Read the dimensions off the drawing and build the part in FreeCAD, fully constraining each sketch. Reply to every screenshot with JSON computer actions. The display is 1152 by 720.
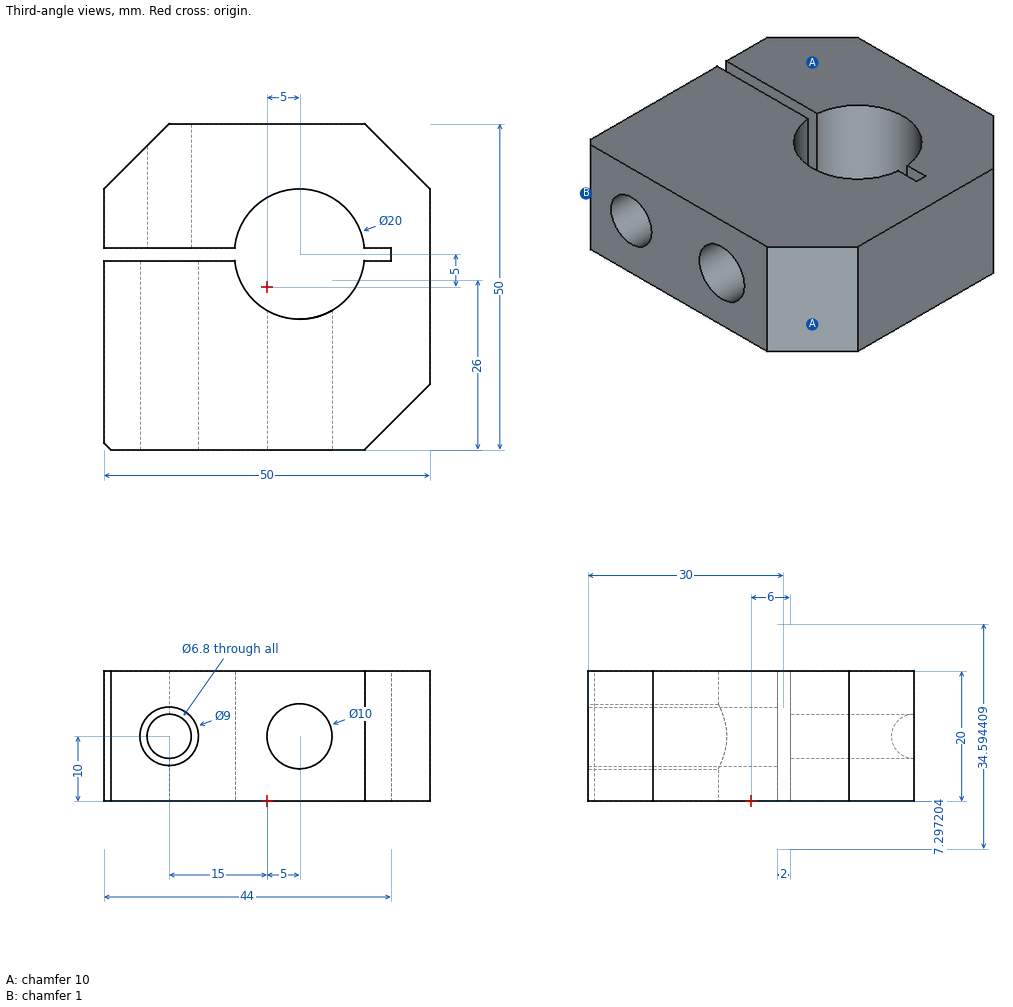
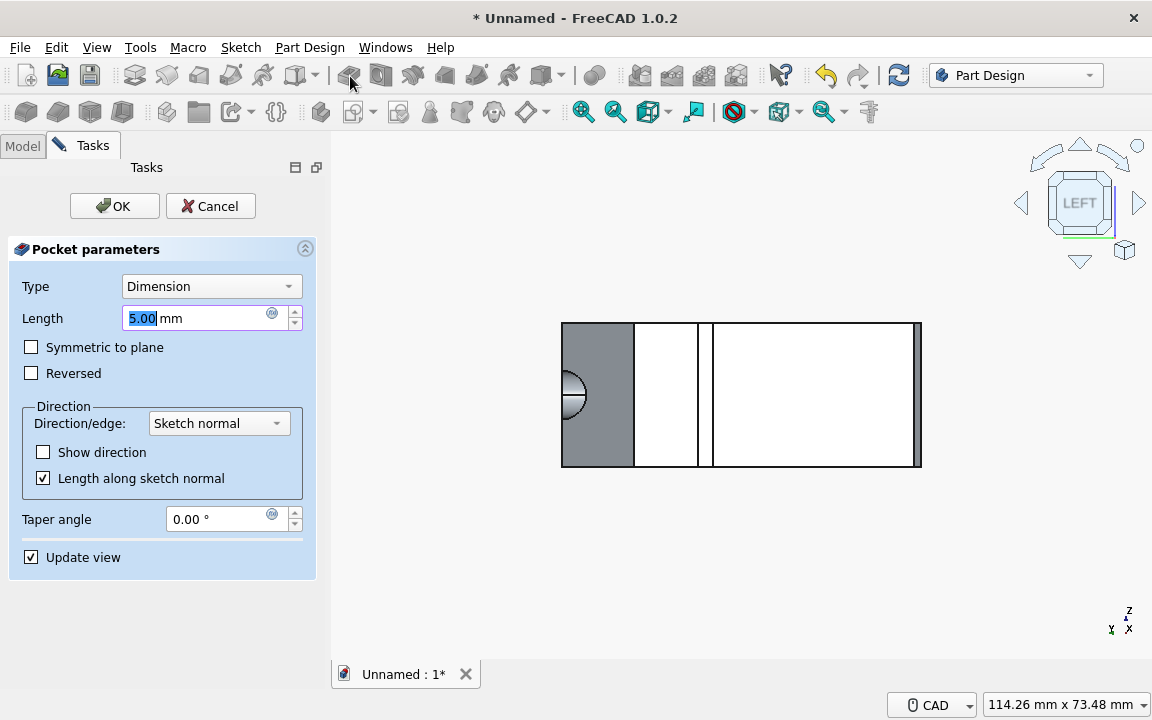
{"action": "type", "text": "44"}
{"action": "key", "text": "Tab"}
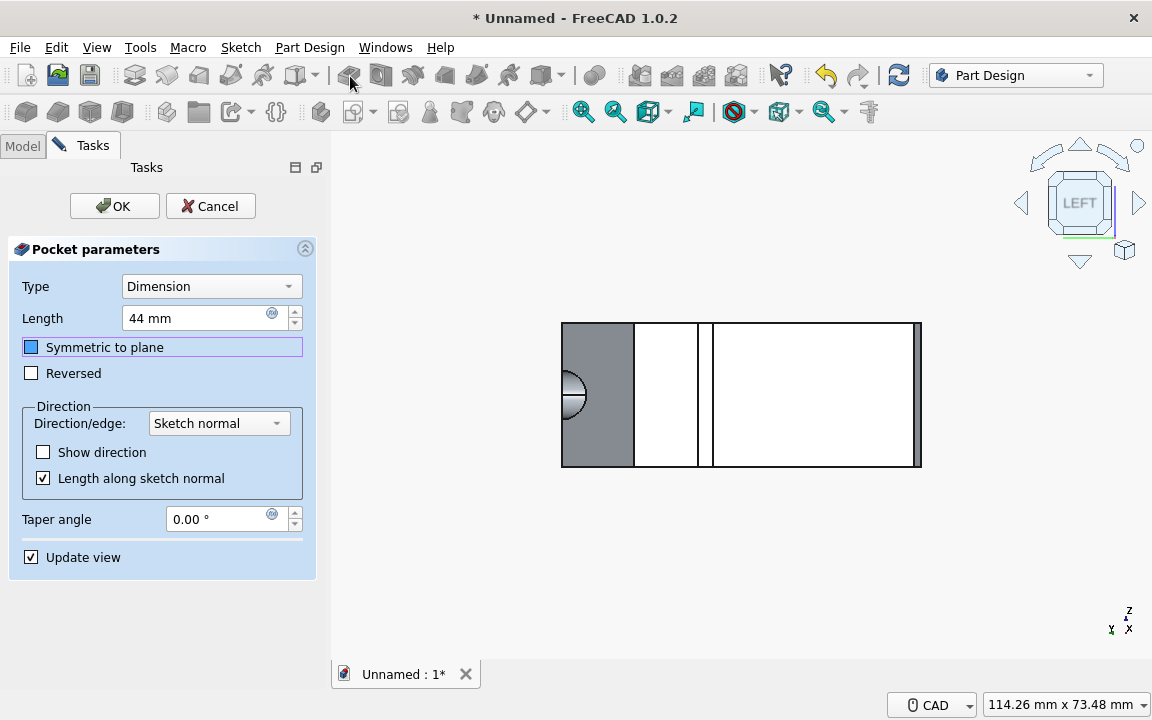
{"action": "left_click", "coordinate": [115, 206]}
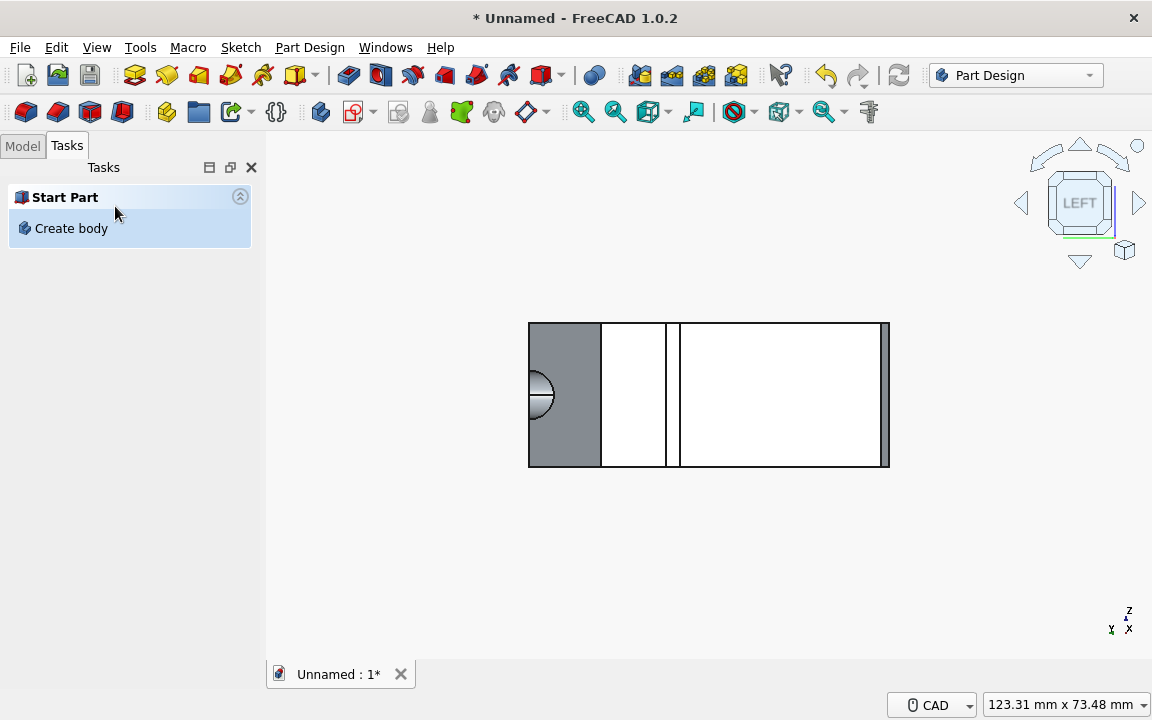
{"action": "left_click", "coordinate": [584, 112]}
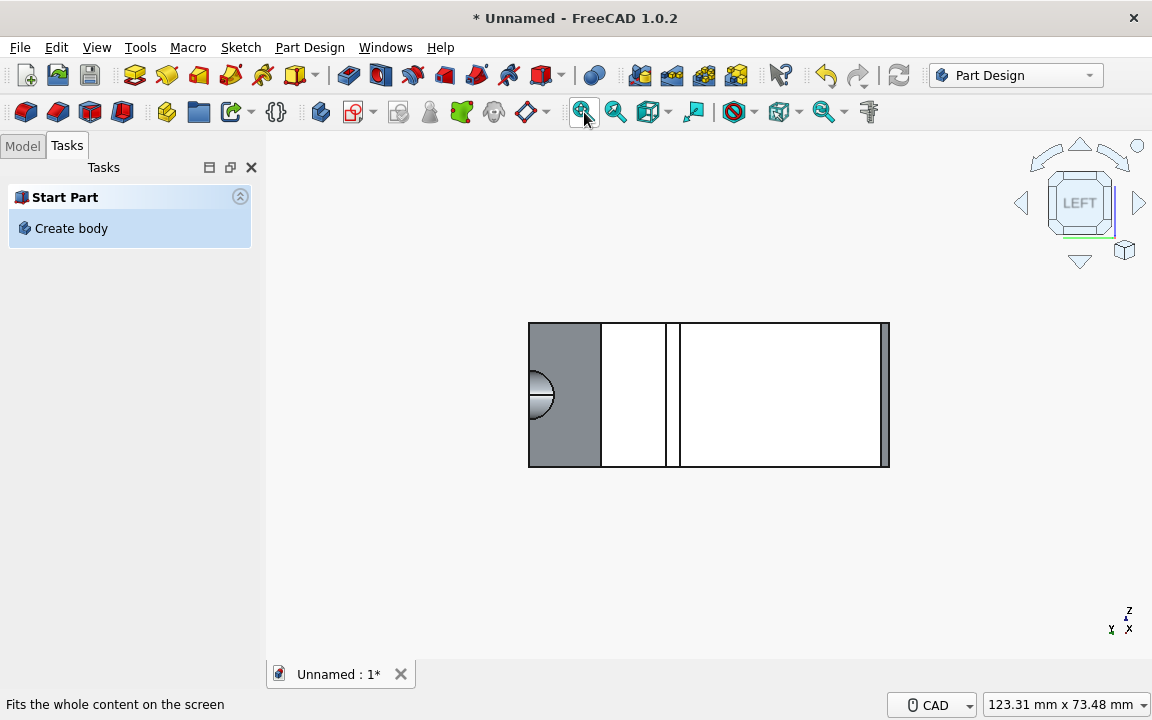
{"action": "key", "text": "0"}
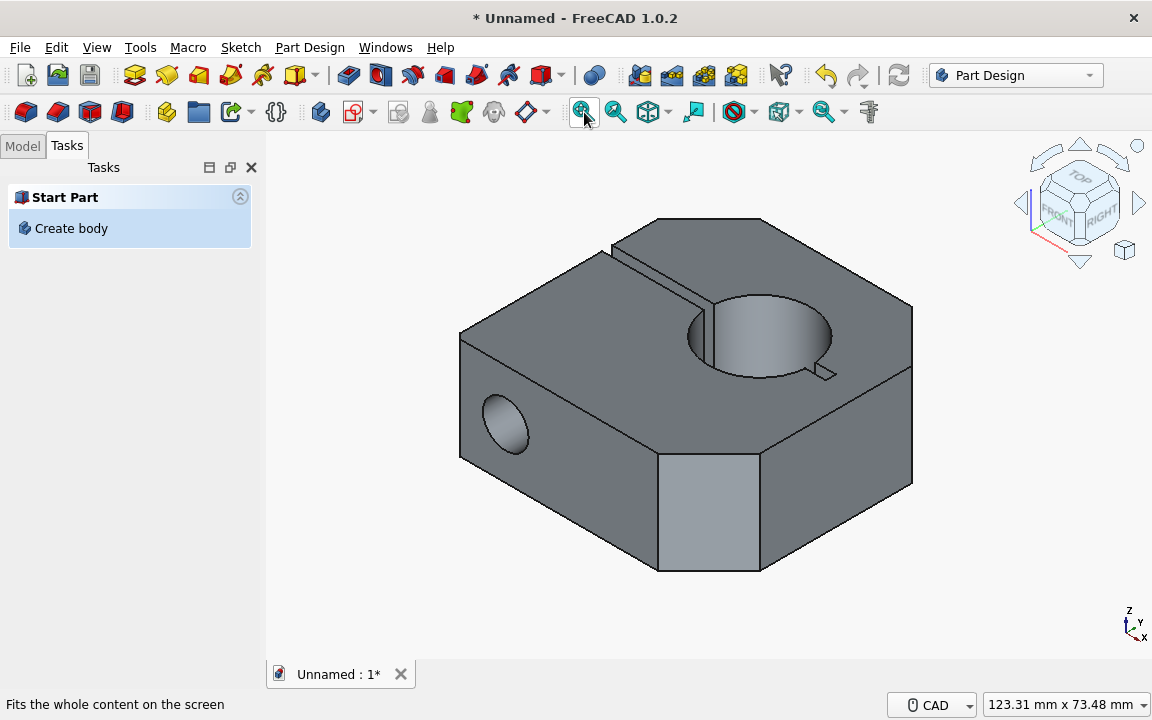
{"action": "left_click", "coordinate": [587, 470]}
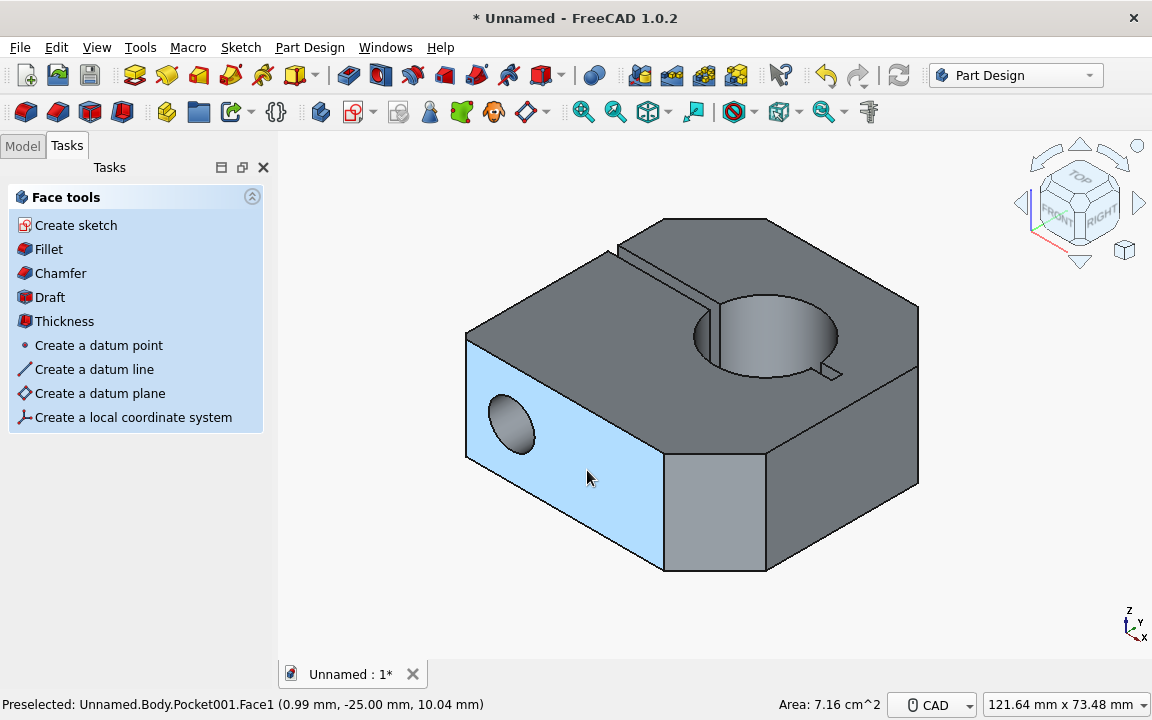
{"action": "left_click", "coordinate": [354, 112]}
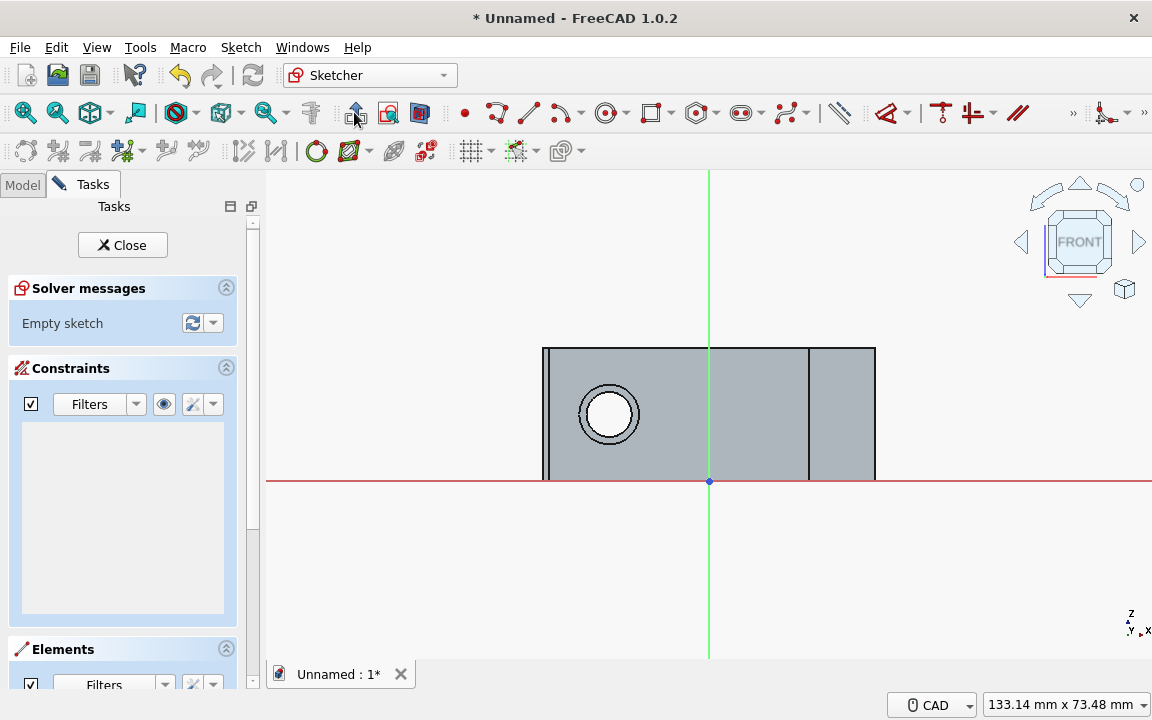
{"action": "scroll", "coordinate": [786, 438], "scroll_direction": "up", "scroll_amount": 6}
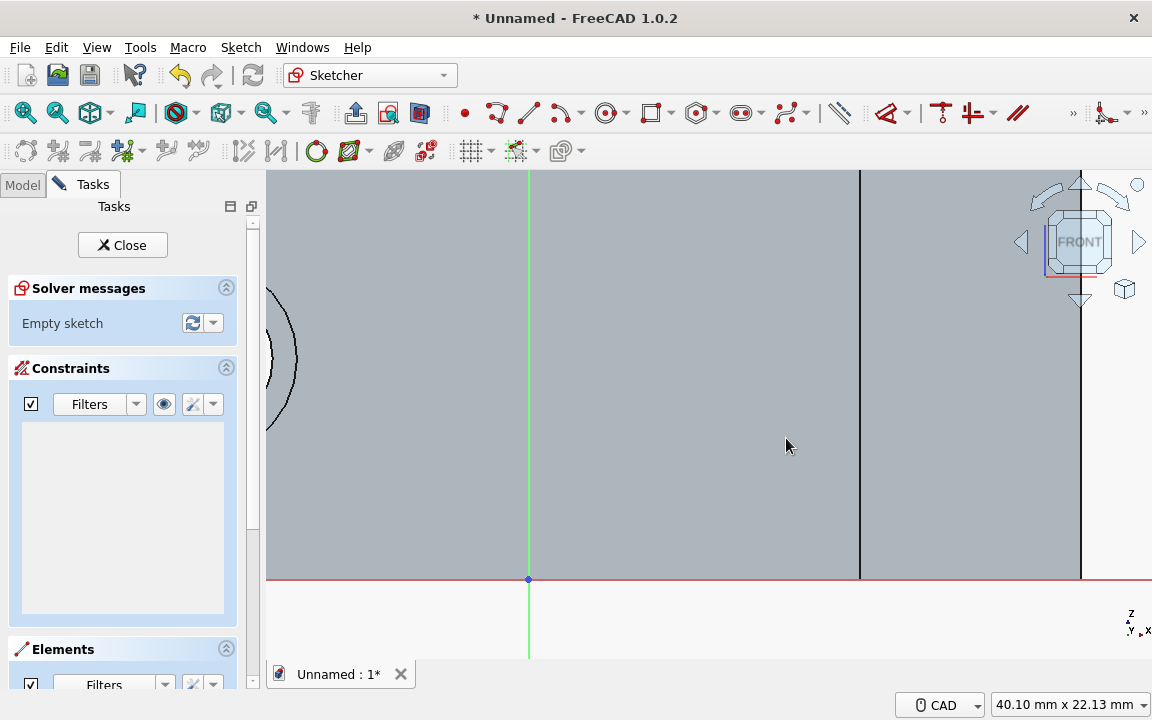
{"action": "left_click", "coordinate": [606, 114]}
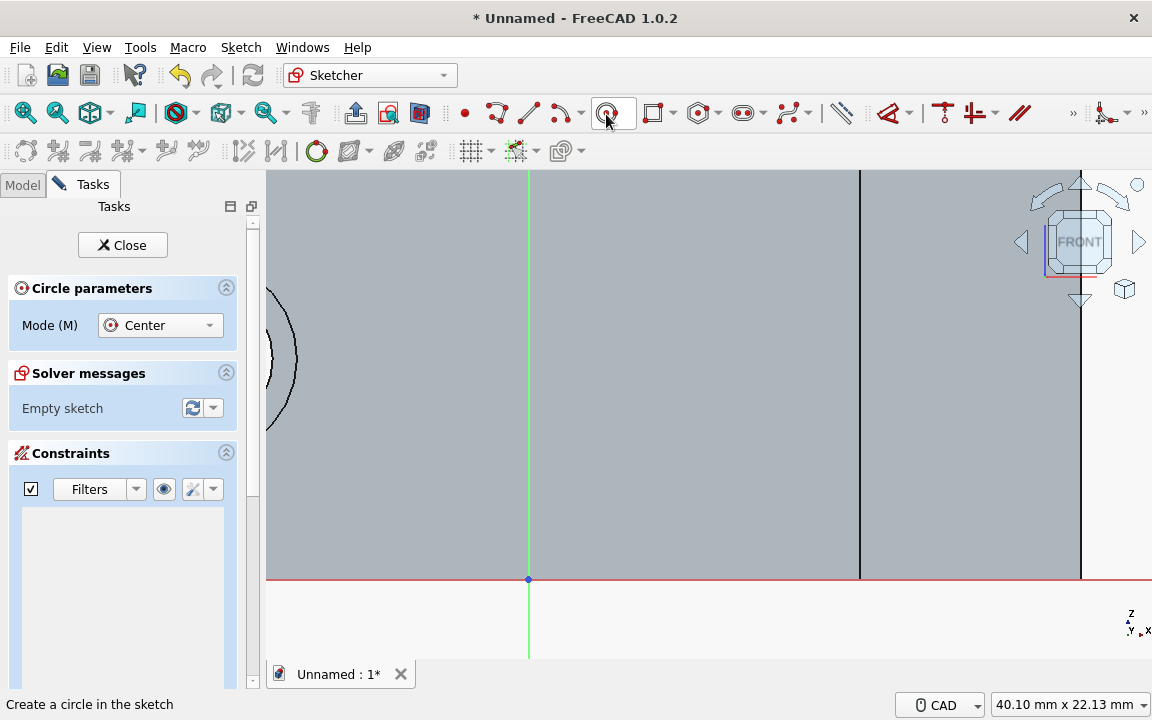
{"action": "left_click", "coordinate": [639, 359]}
{"action": "mouse_move", "coordinate": [718, 281]}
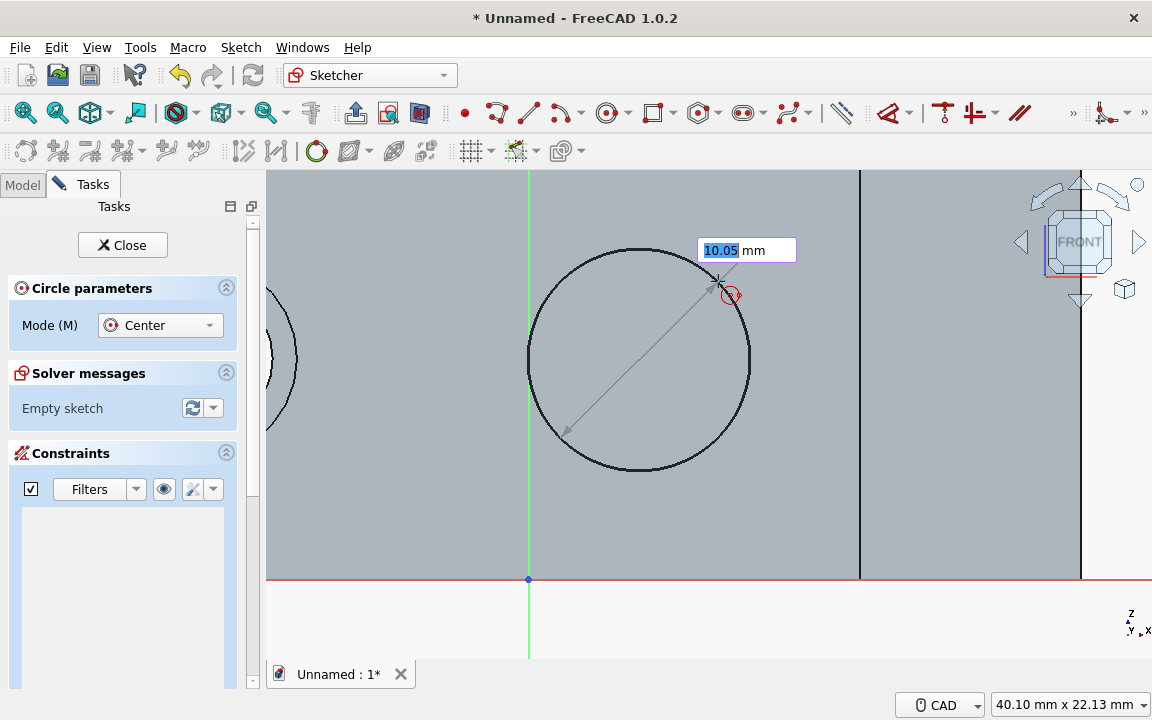
{"action": "type", "text": "10"}
{"action": "key", "text": "Return"}
{"action": "key", "text": "Escape"}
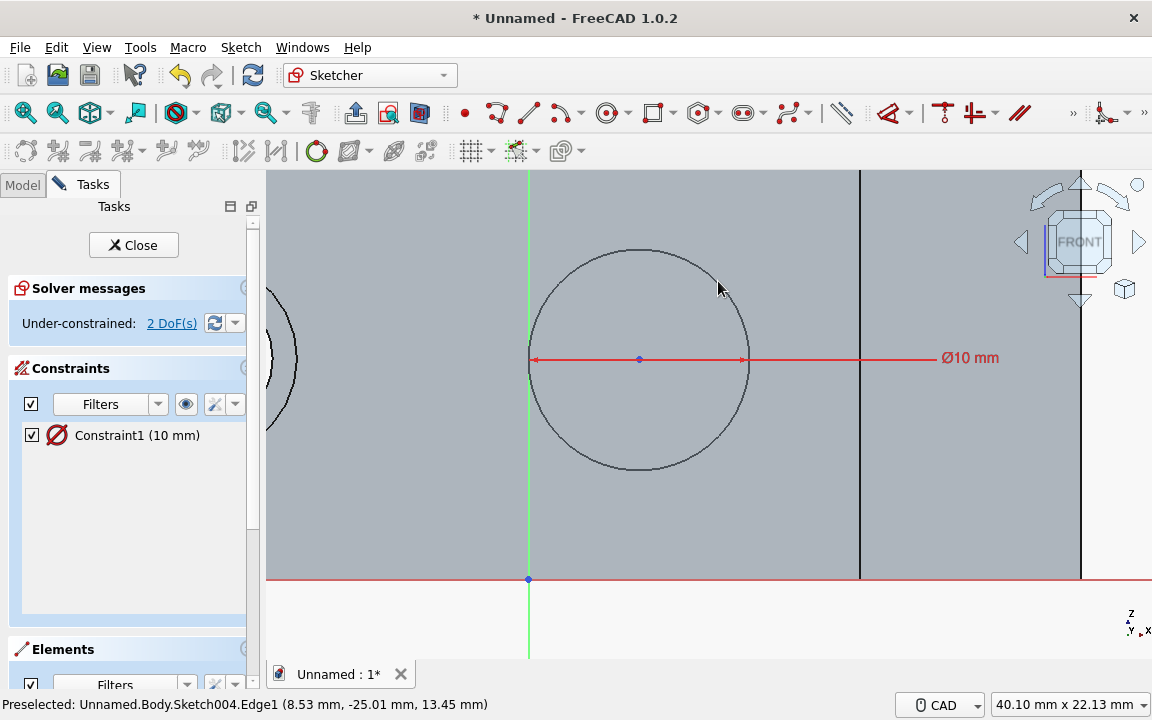
{"action": "left_click", "coordinate": [888, 114]}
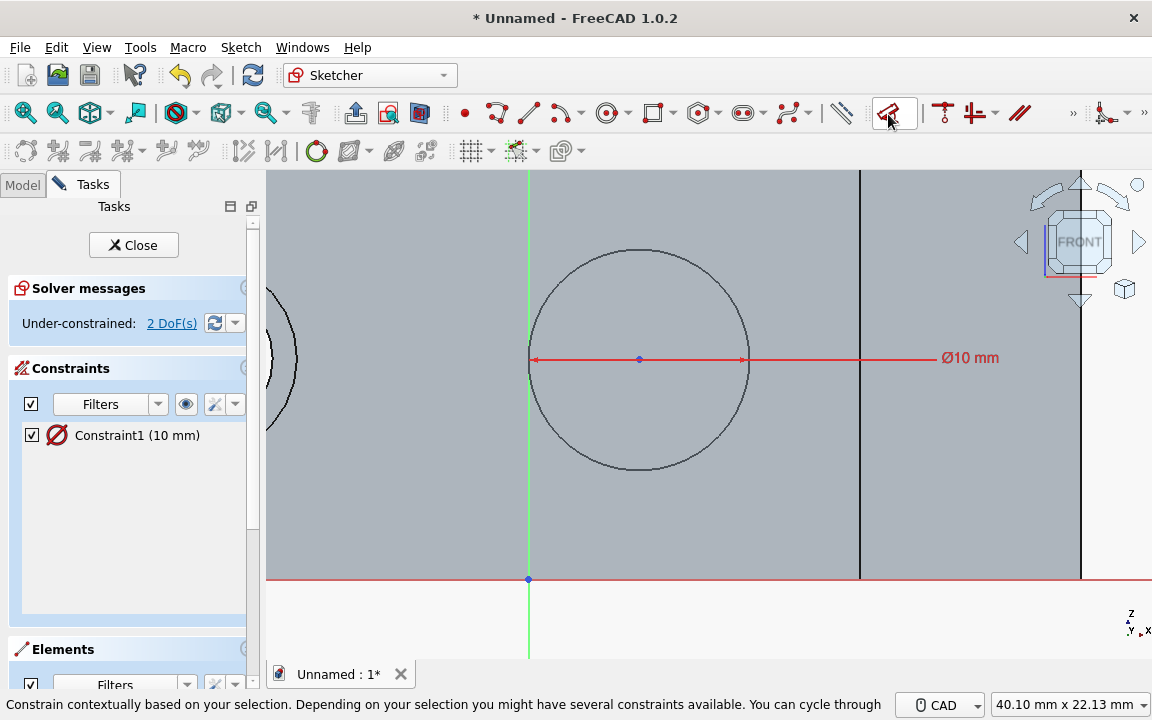
{"action": "left_click", "coordinate": [639, 360]}
{"action": "left_click", "coordinate": [584, 614]}